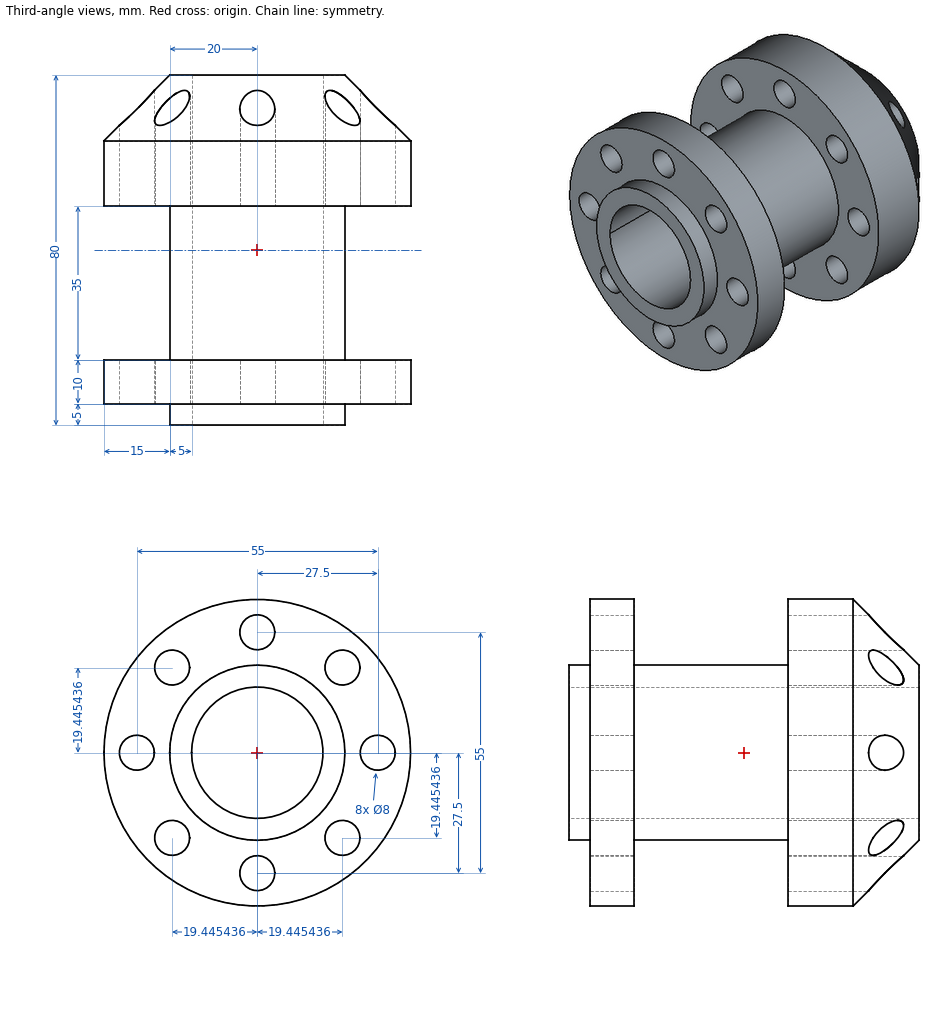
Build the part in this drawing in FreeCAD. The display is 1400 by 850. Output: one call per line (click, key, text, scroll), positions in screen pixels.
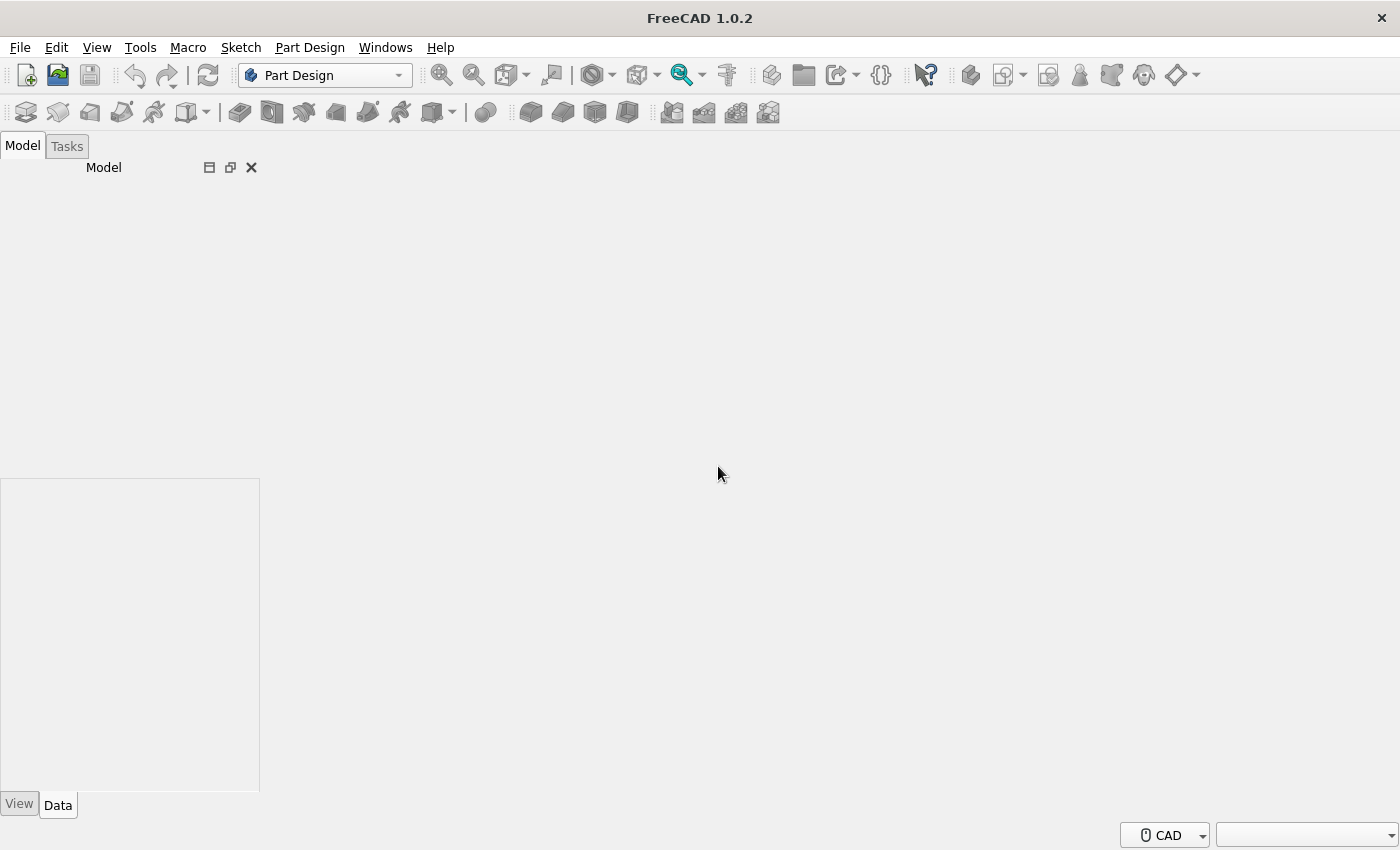
key(ctrl+n)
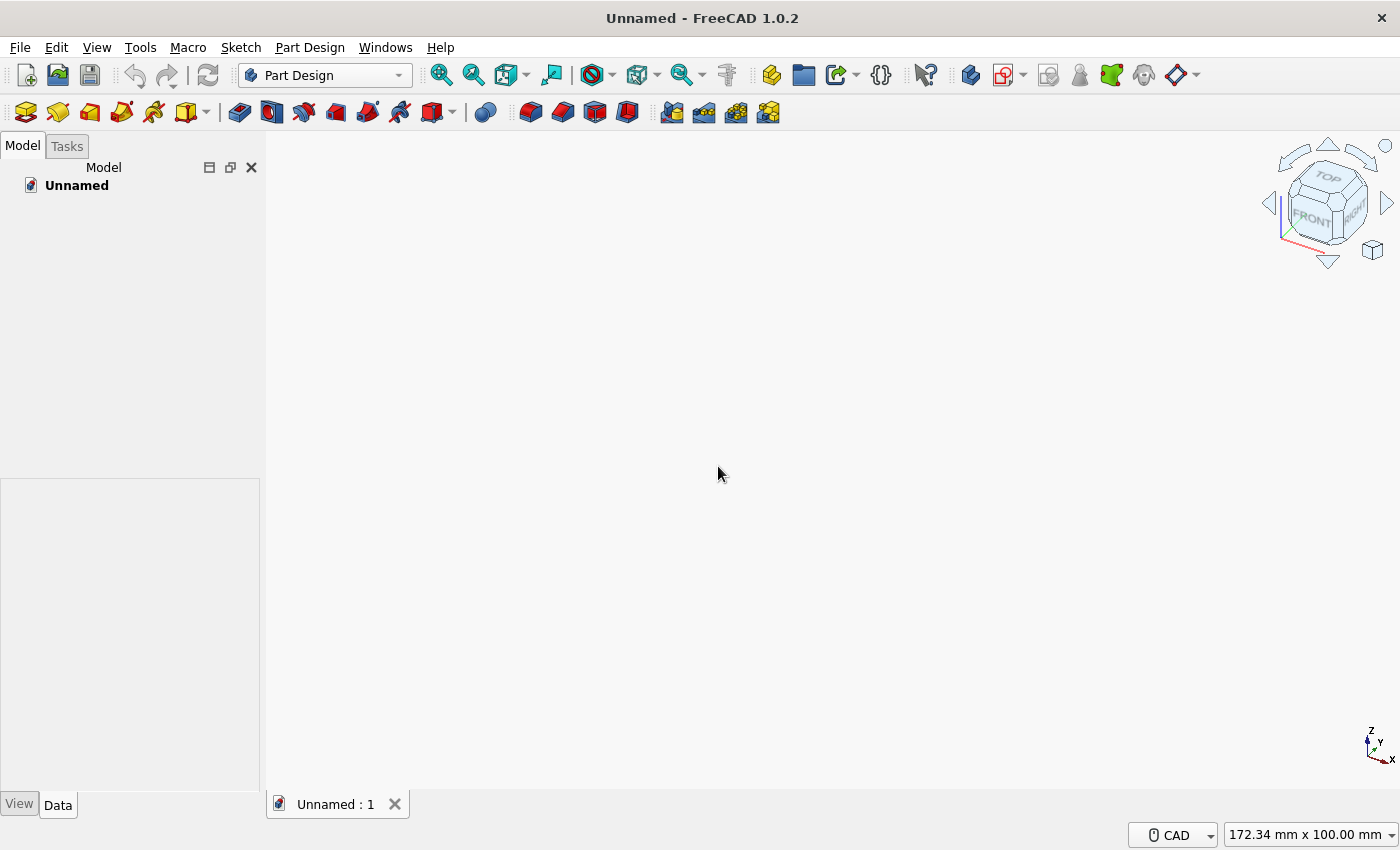
click(1004, 76)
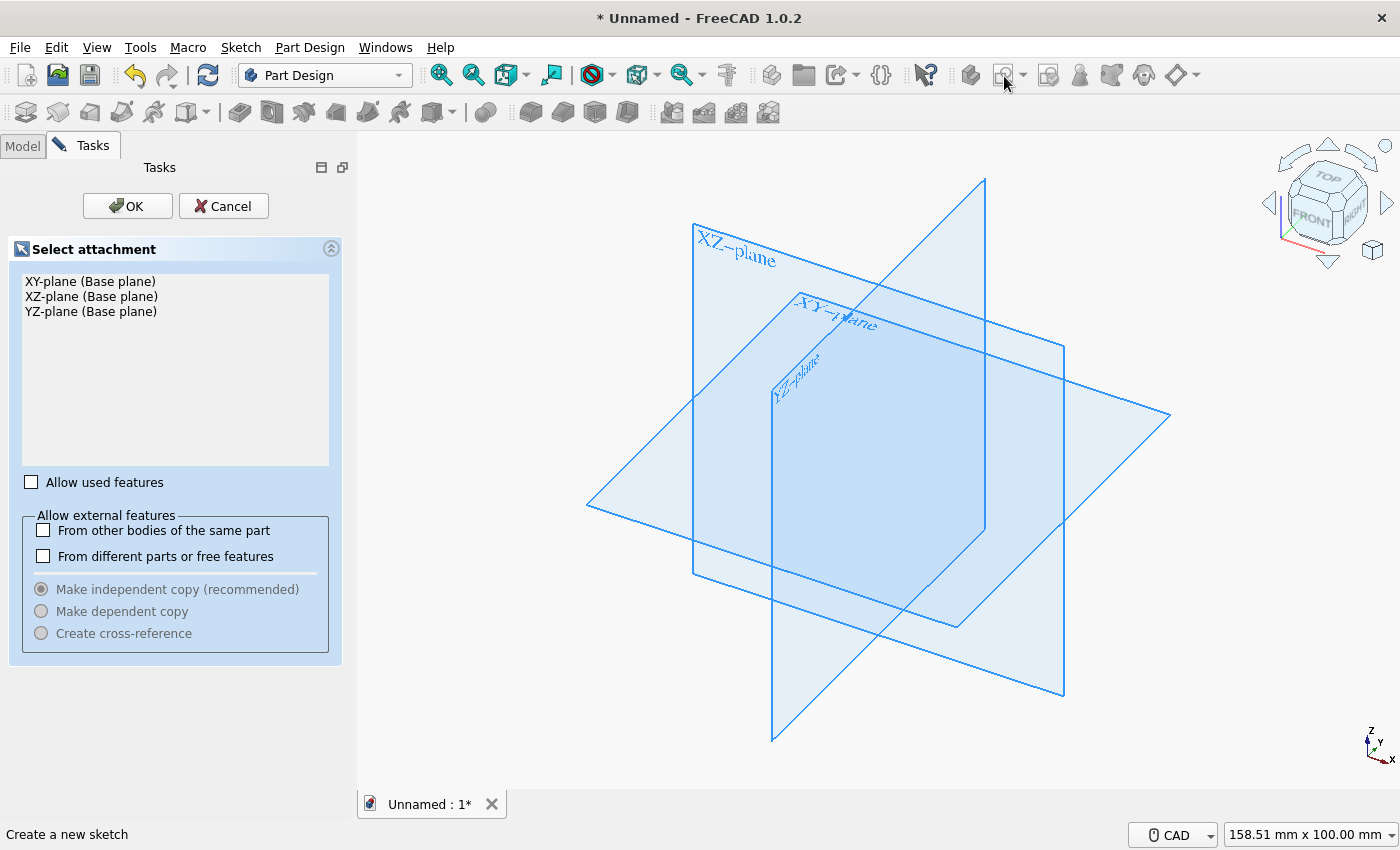
click(82, 282)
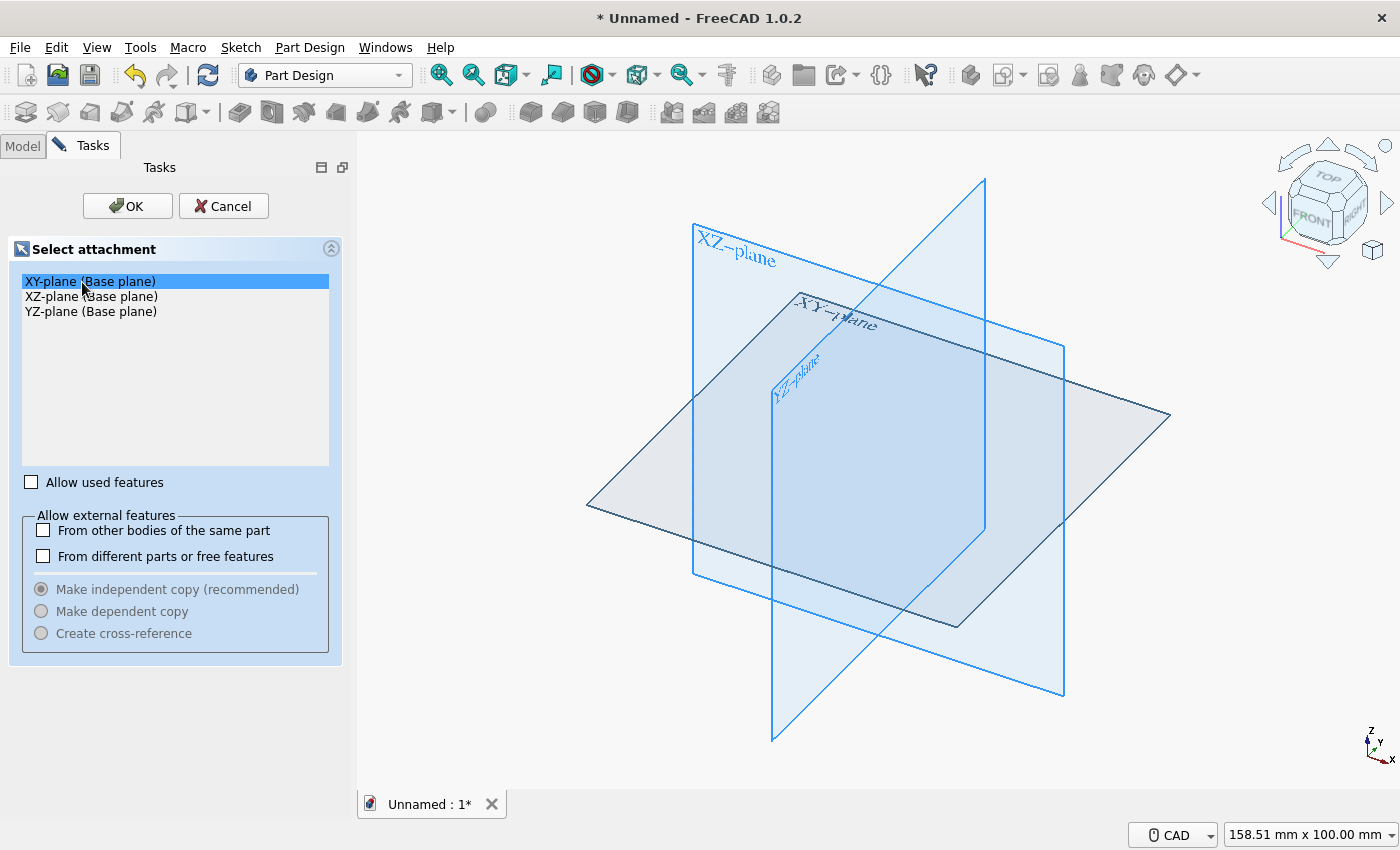
click(128, 206)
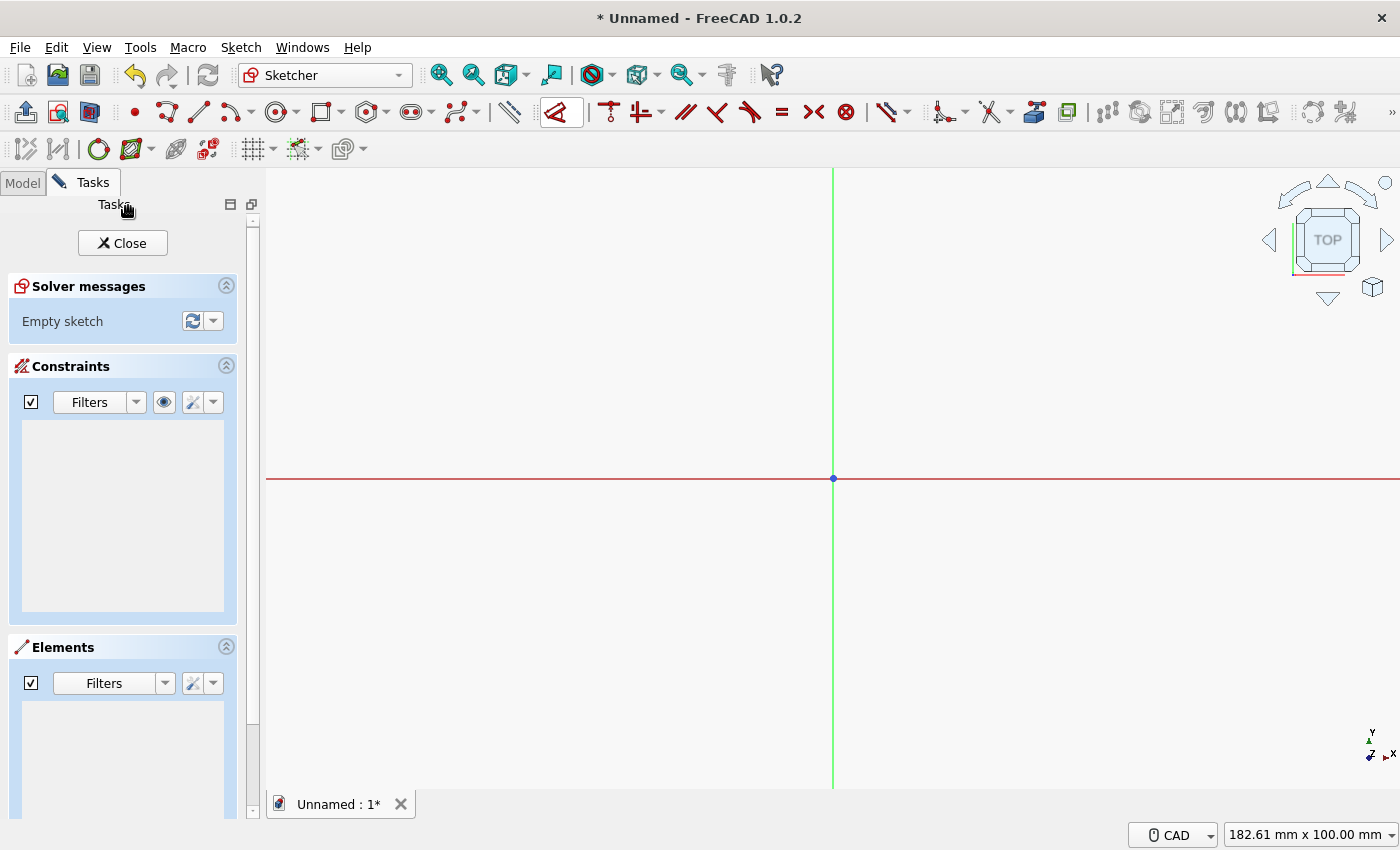
key(g)
key(m)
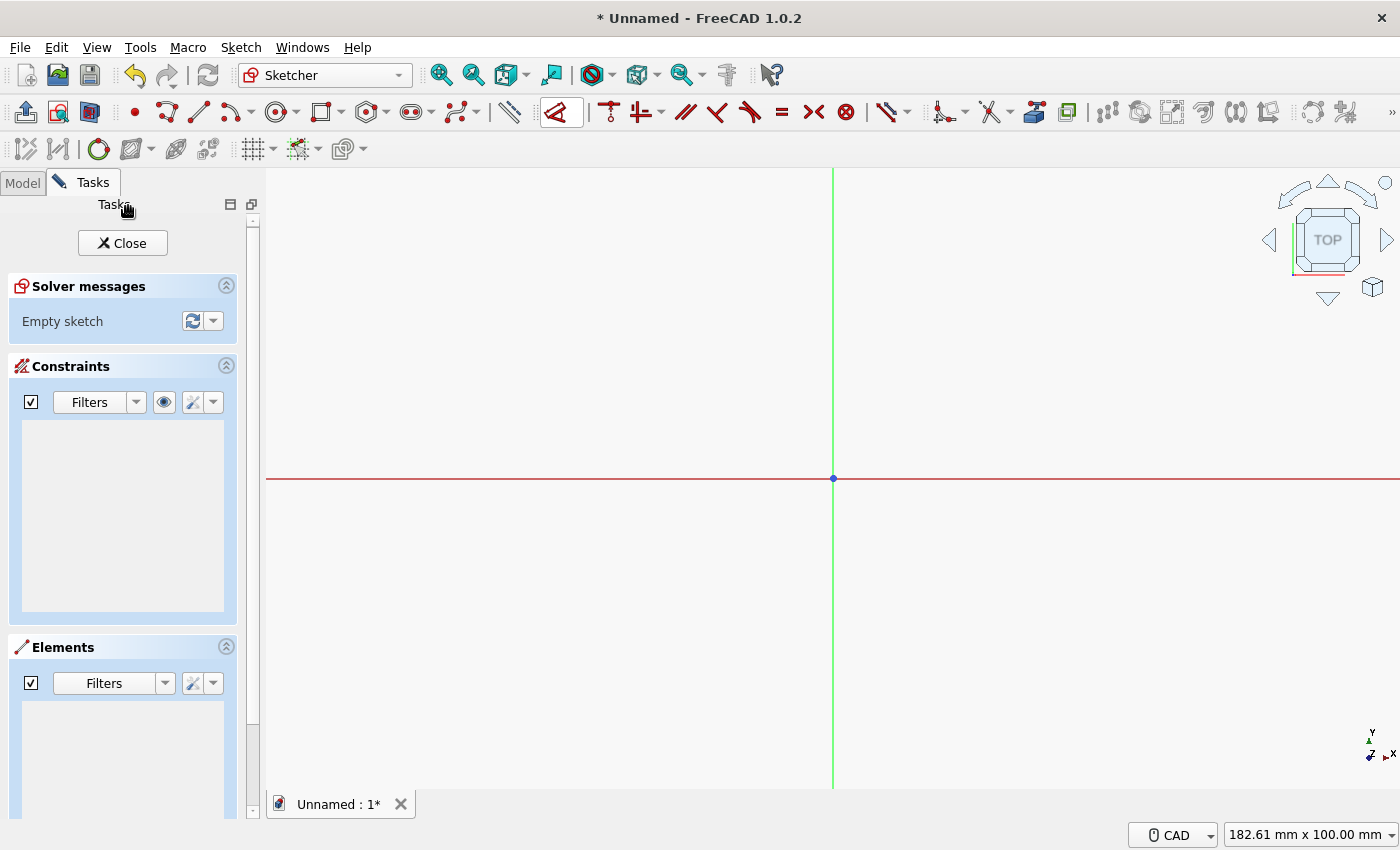
click(709, 416)
click(709, 634)
click(616, 634)
click(616, 696)
click(709, 696)
click(709, 727)
click(740, 727)
click(740, 230)
click(709, 230)
click(616, 323)
click(616, 416)
click(709, 417)
key(Escape)
key(Escape)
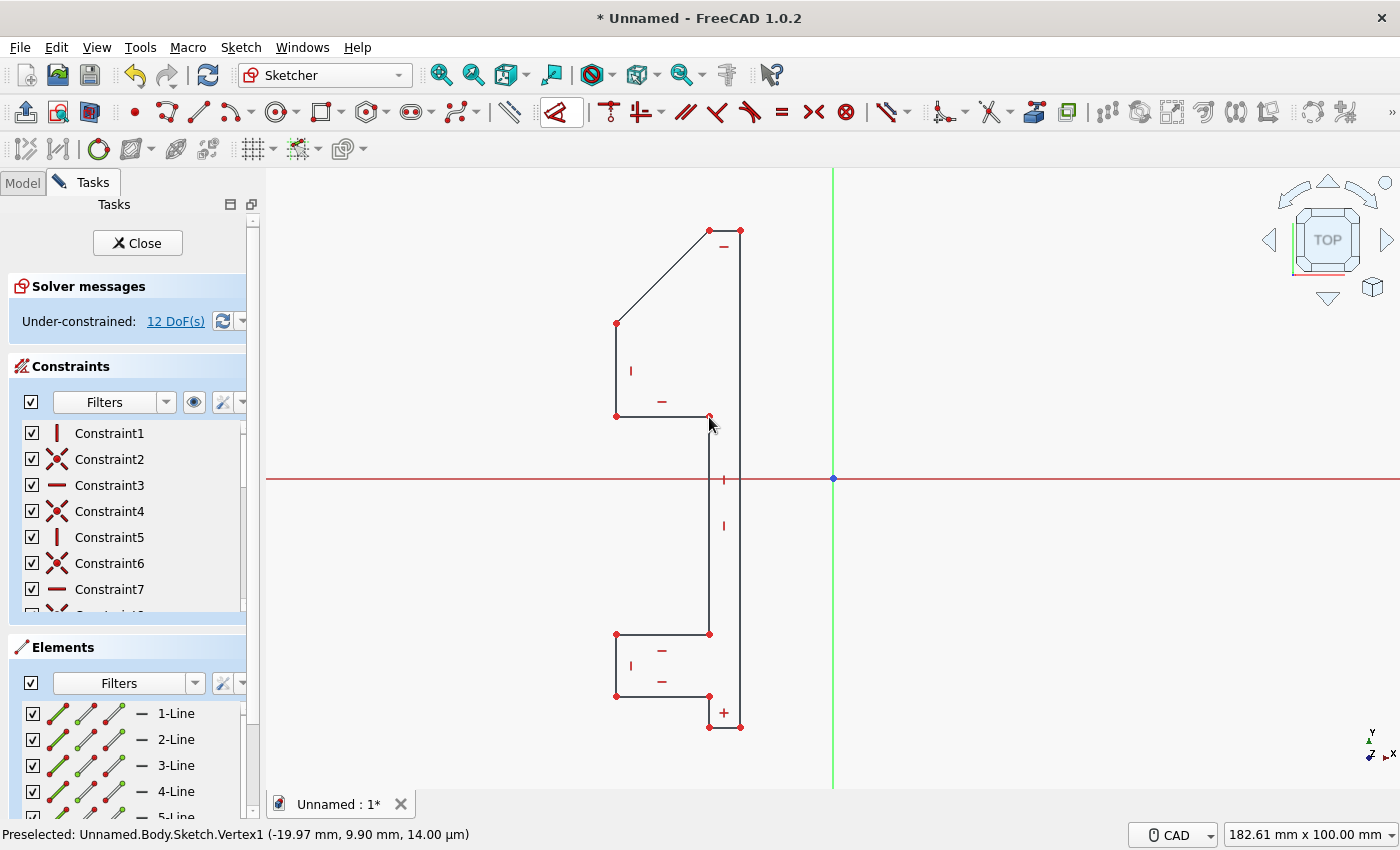
click(709, 728)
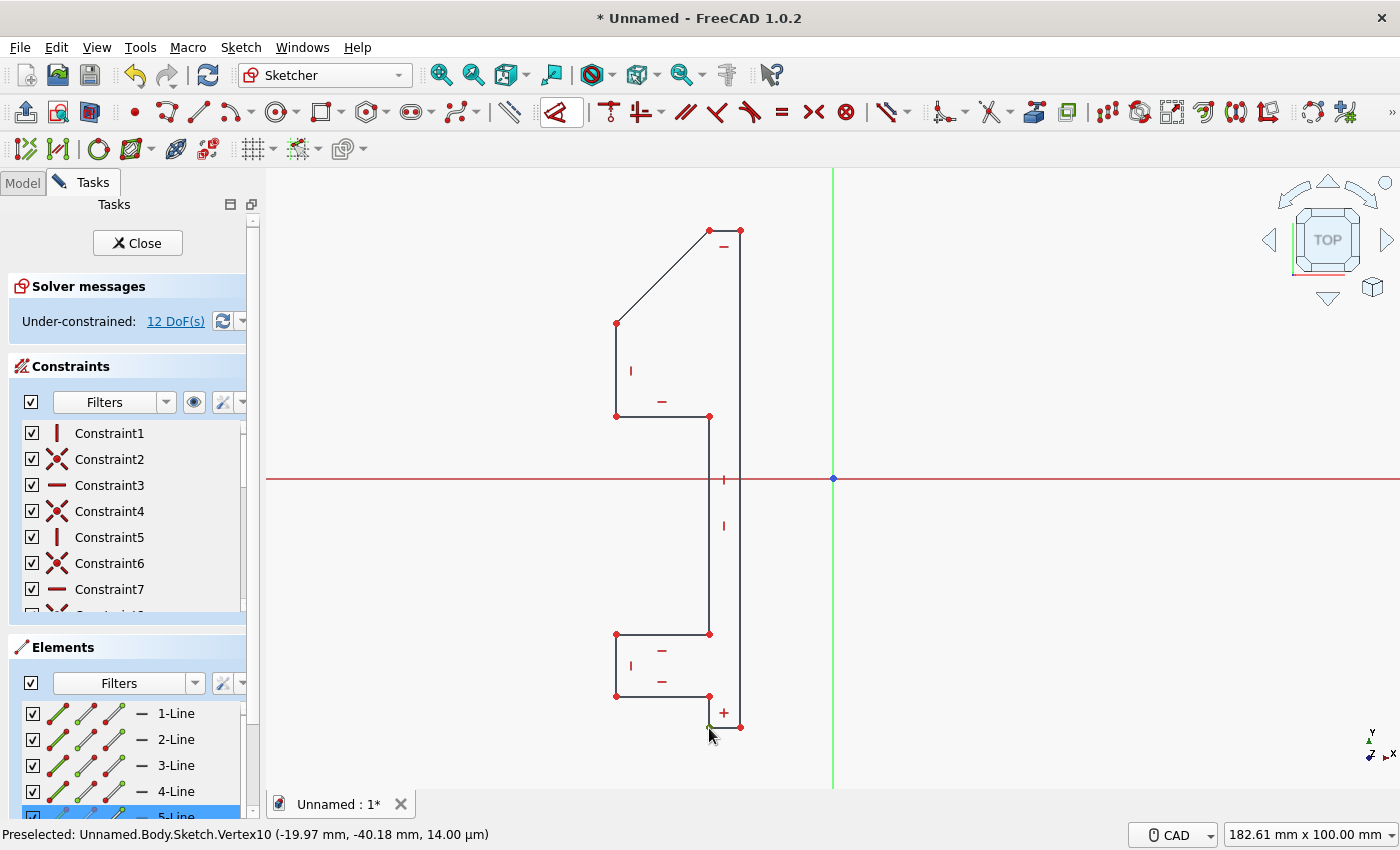
click(709, 231)